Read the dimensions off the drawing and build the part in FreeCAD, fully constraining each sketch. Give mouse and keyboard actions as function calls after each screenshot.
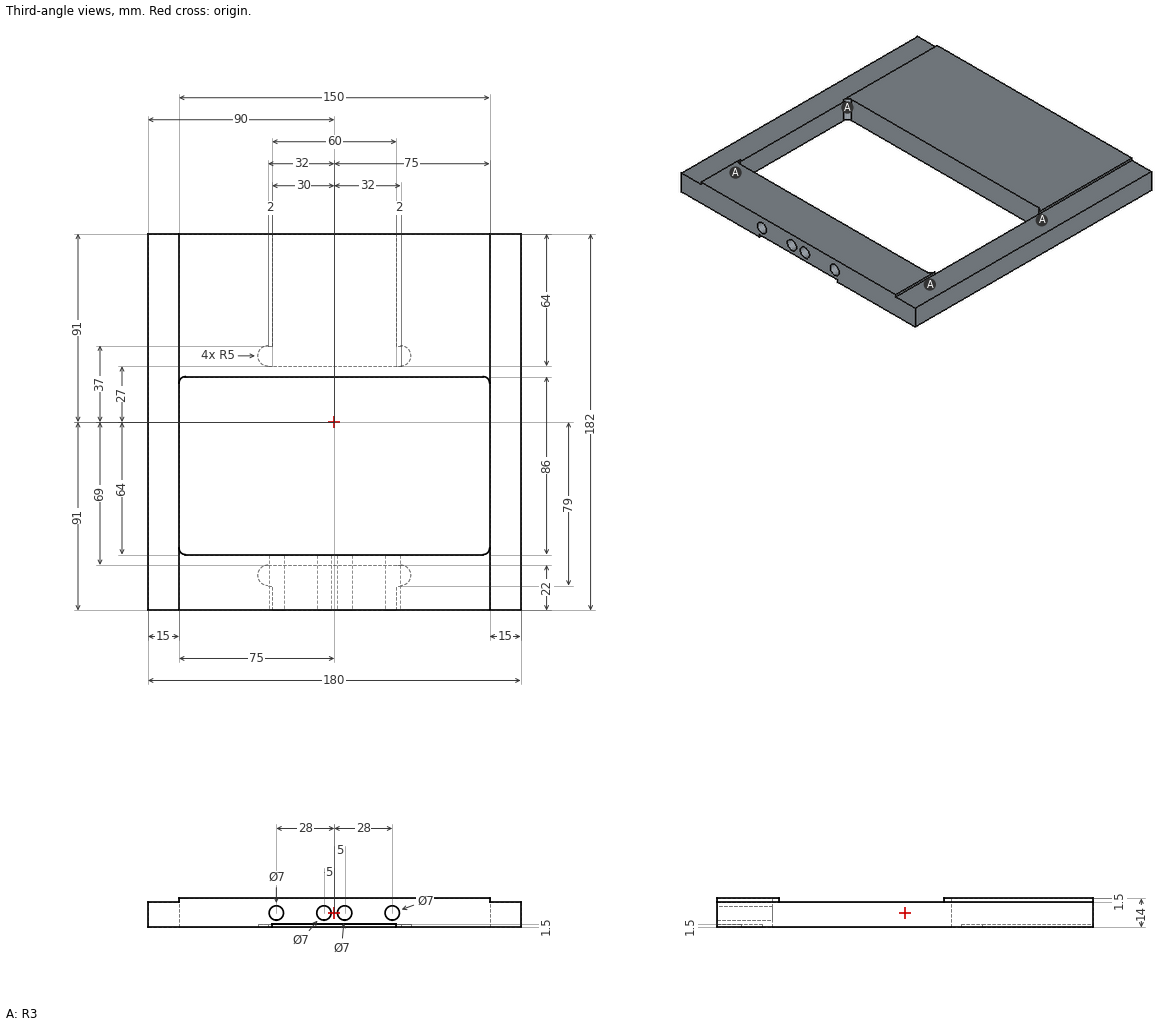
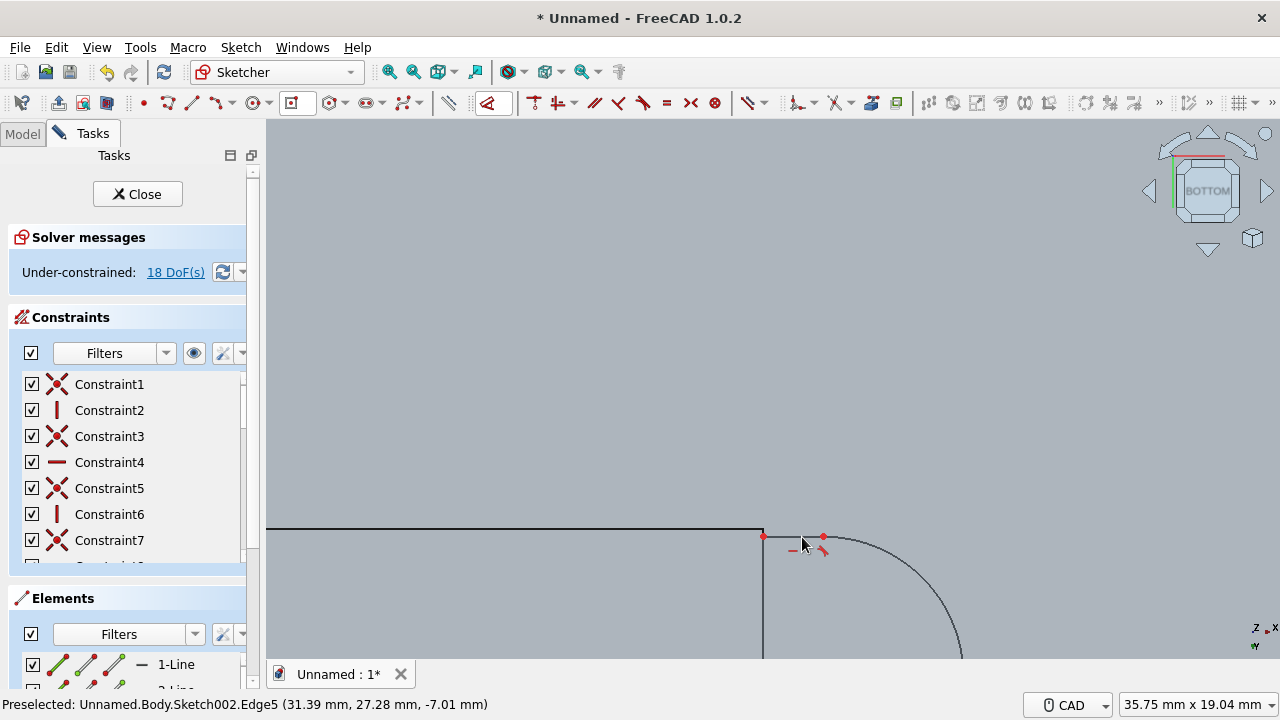
scroll(803, 541, down, 11)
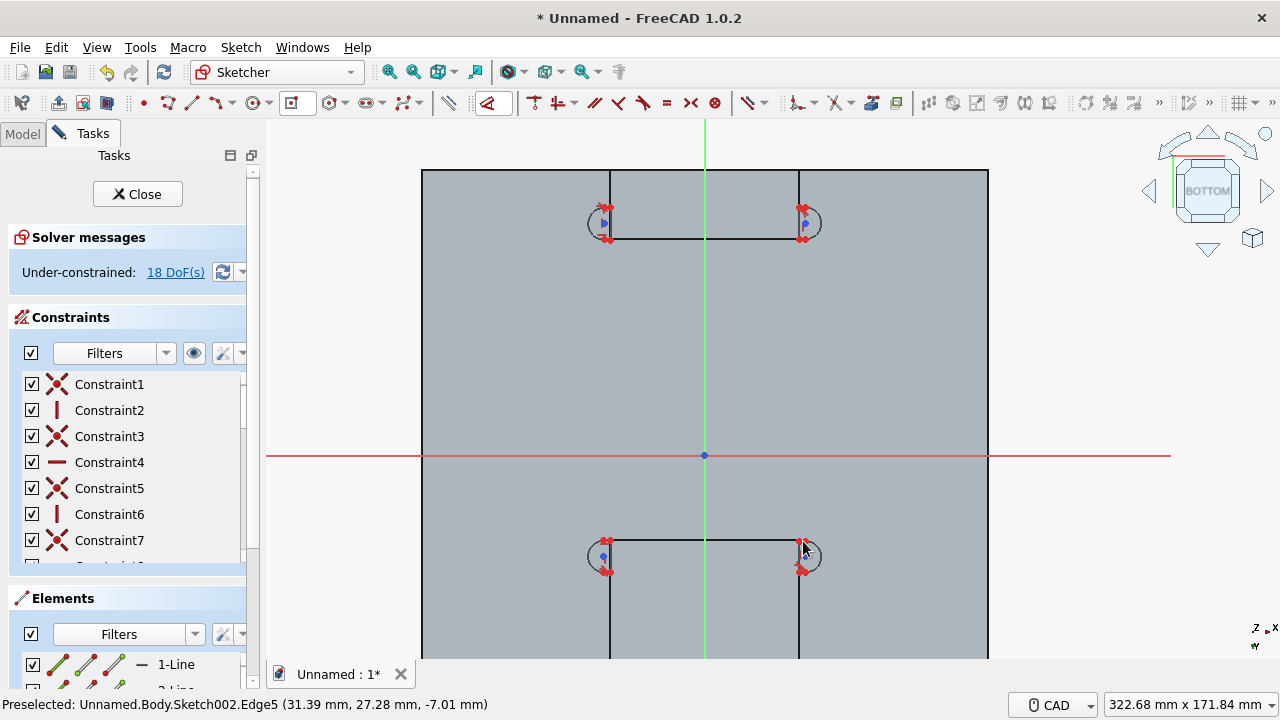
scroll(606, 240, up, 10)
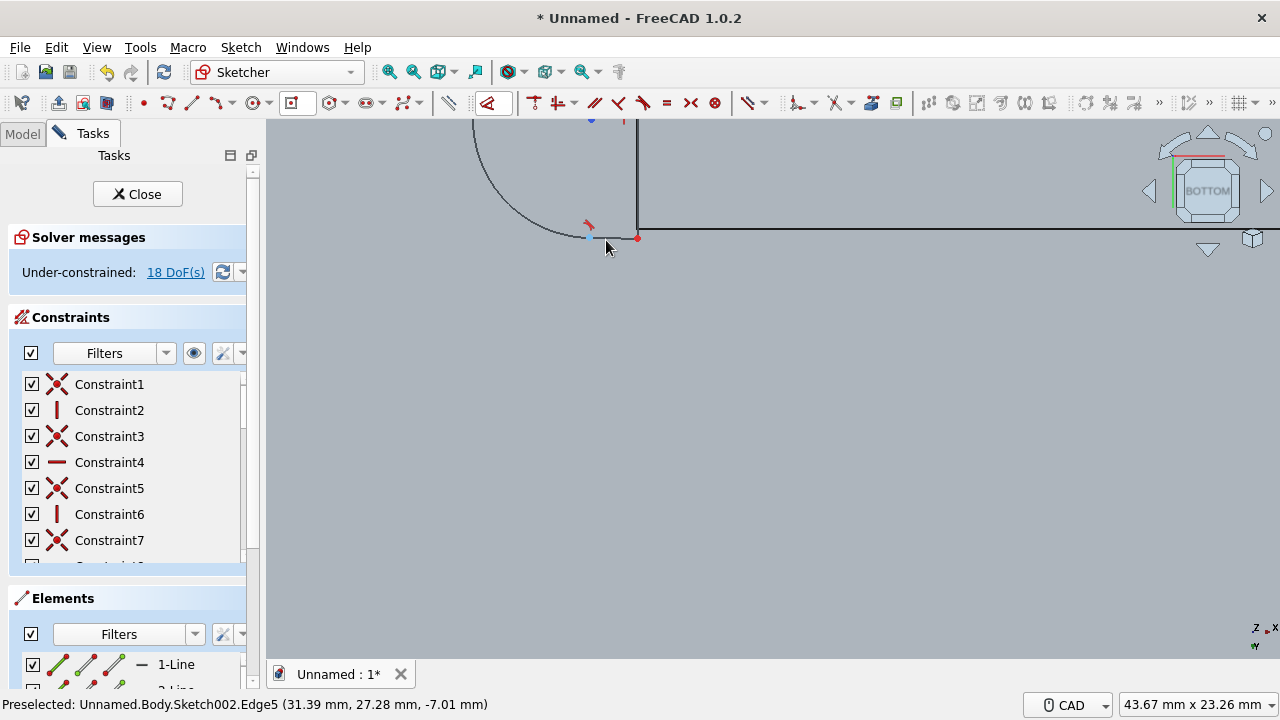
click(604, 238)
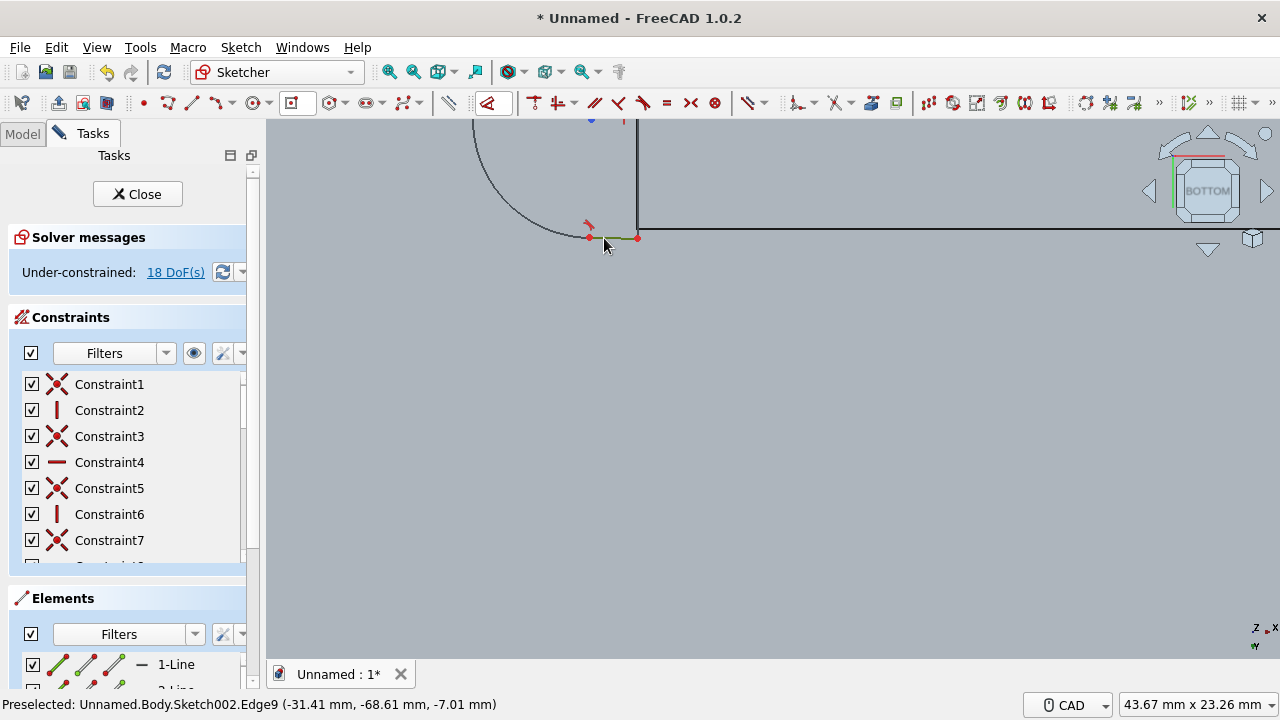
key(h)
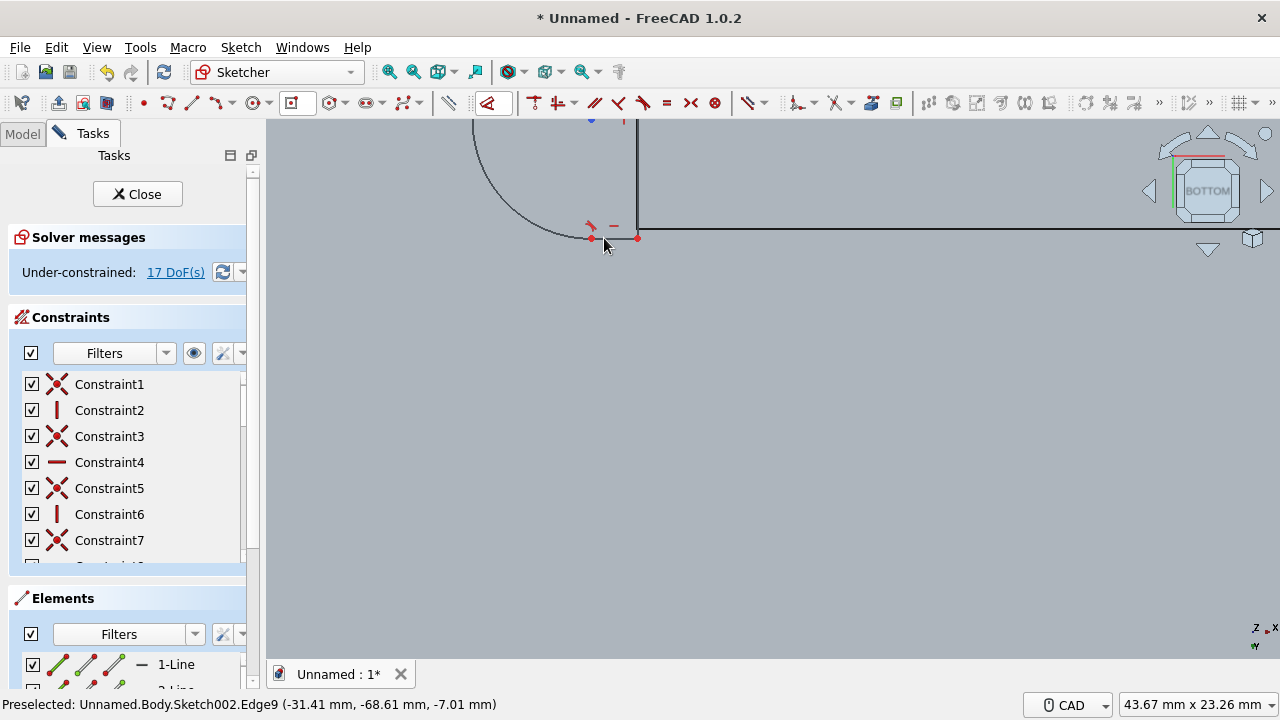
scroll(606, 240, down, 10)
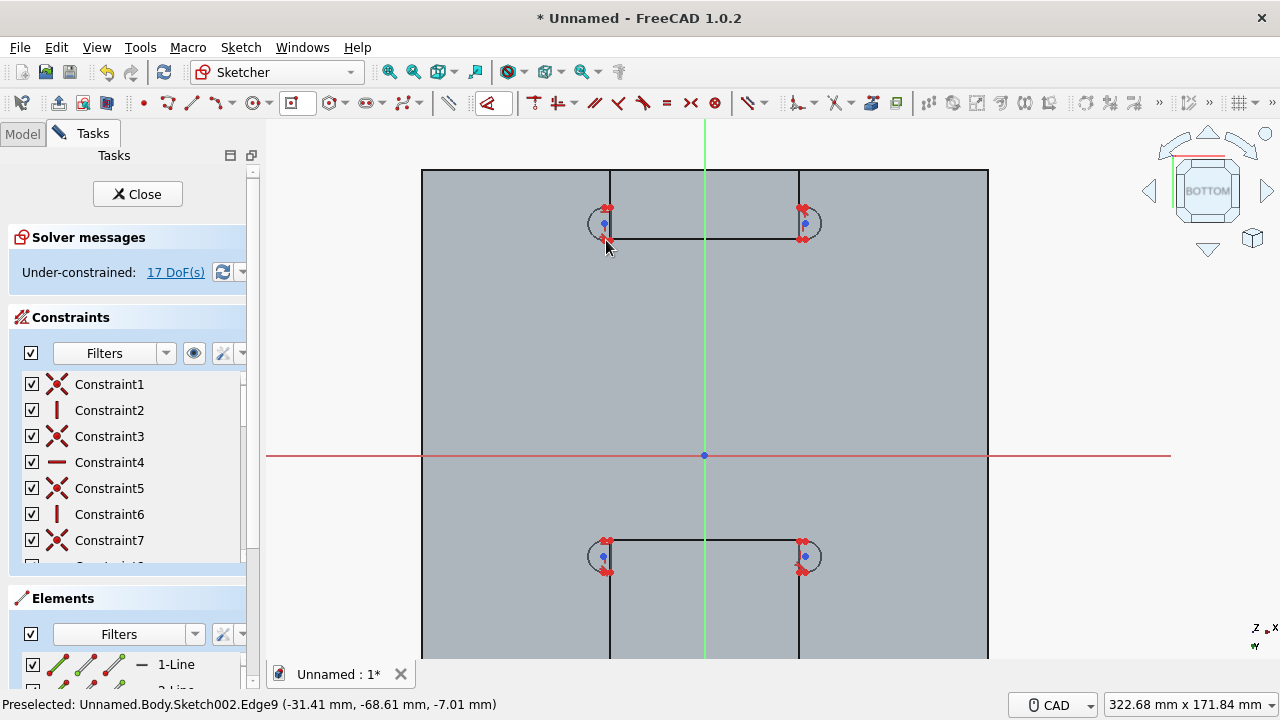
scroll(803, 208, up, 11)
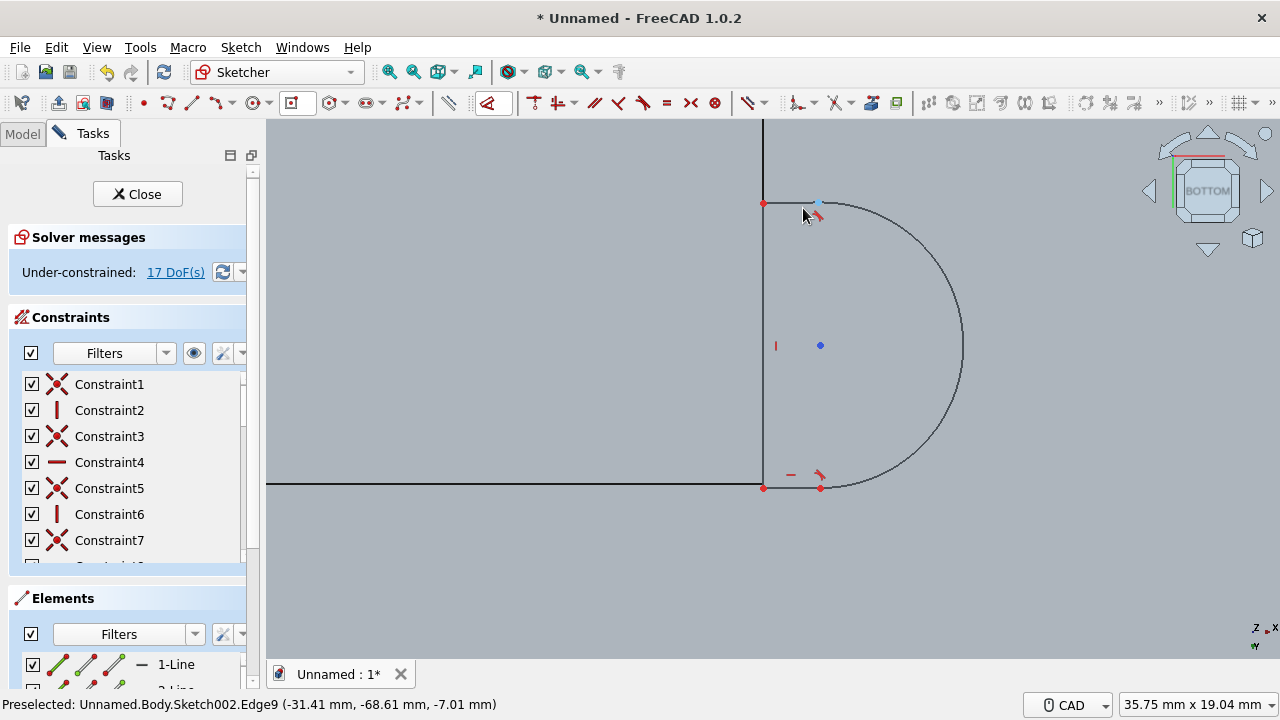
click(802, 203)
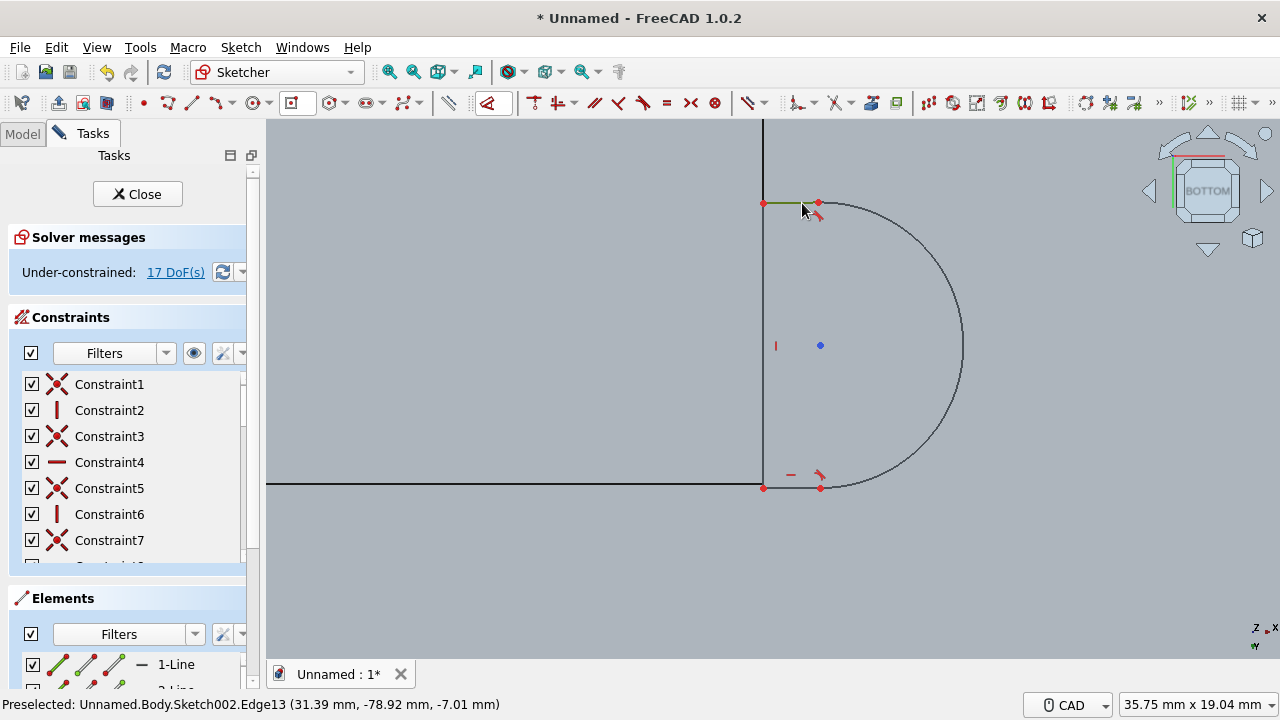
key(h)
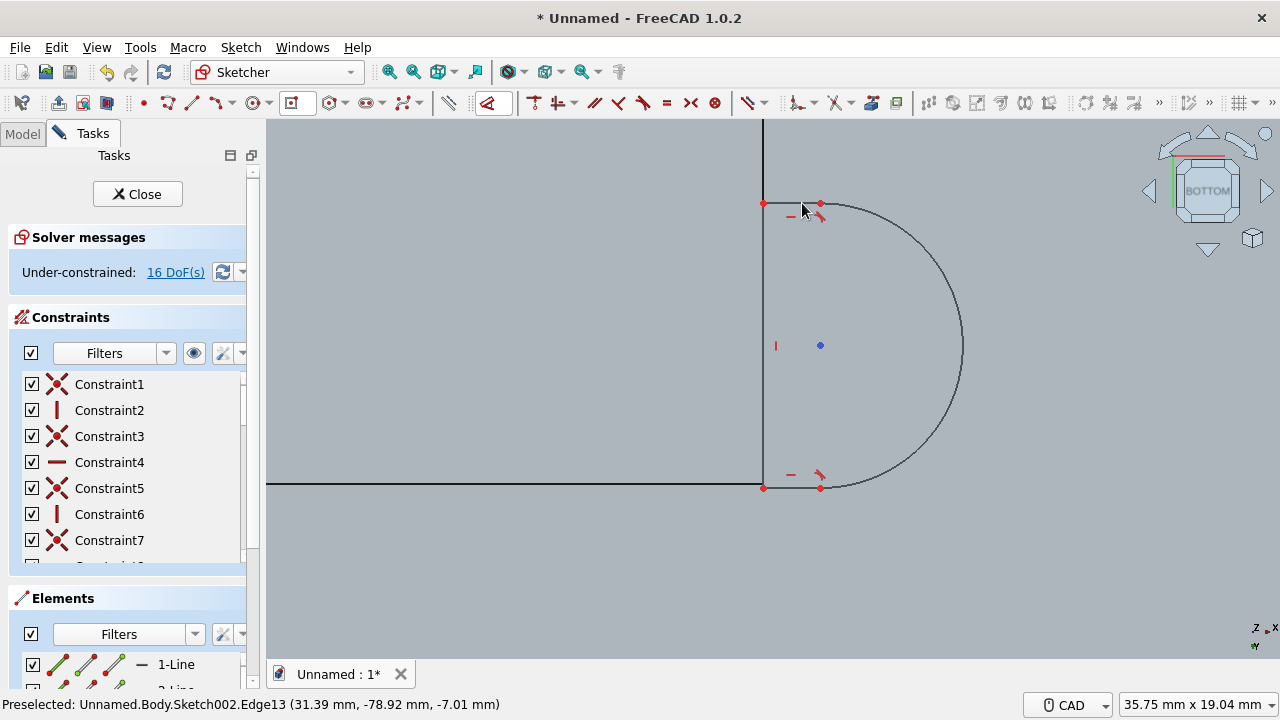
scroll(803, 208, down, 11)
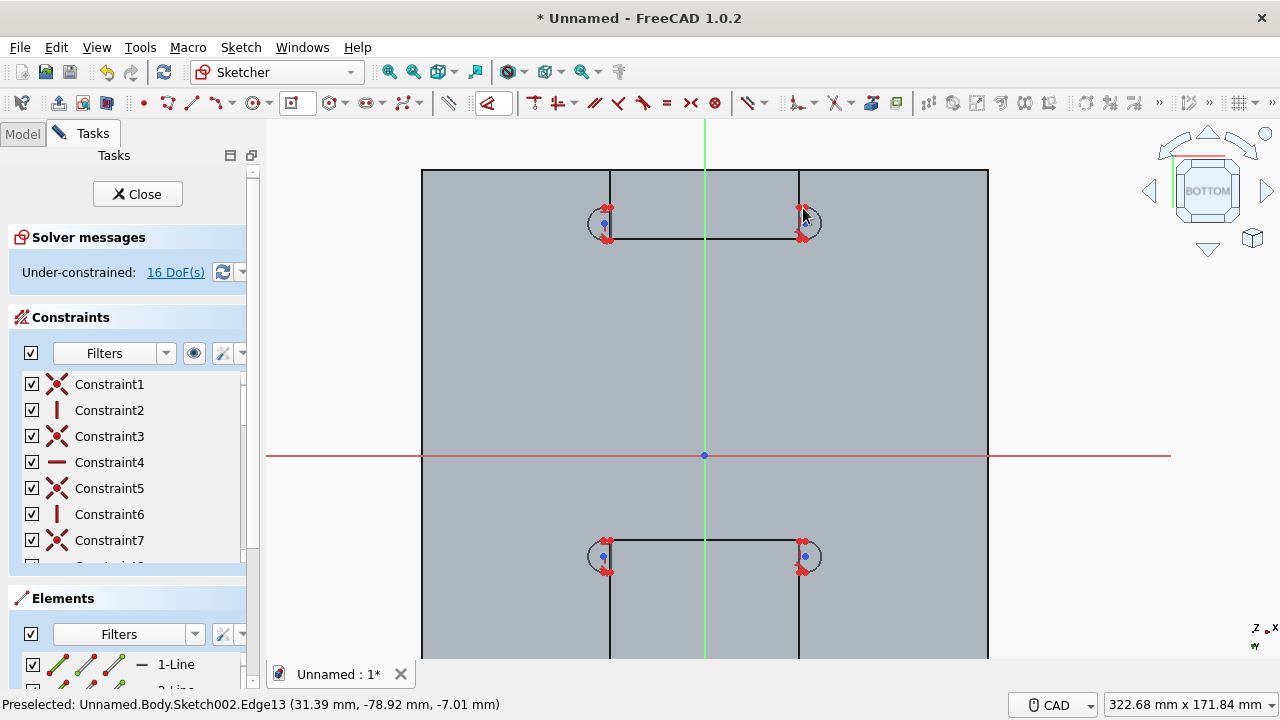
click(591, 547)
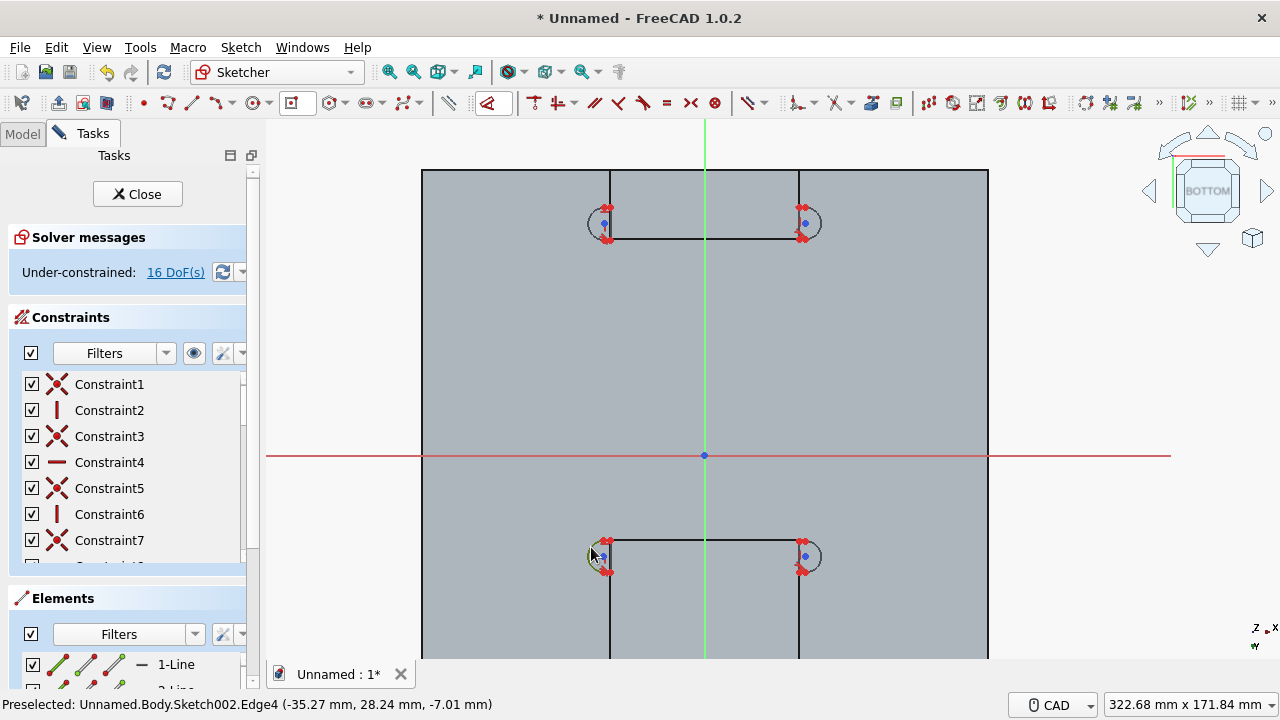
click(818, 566)